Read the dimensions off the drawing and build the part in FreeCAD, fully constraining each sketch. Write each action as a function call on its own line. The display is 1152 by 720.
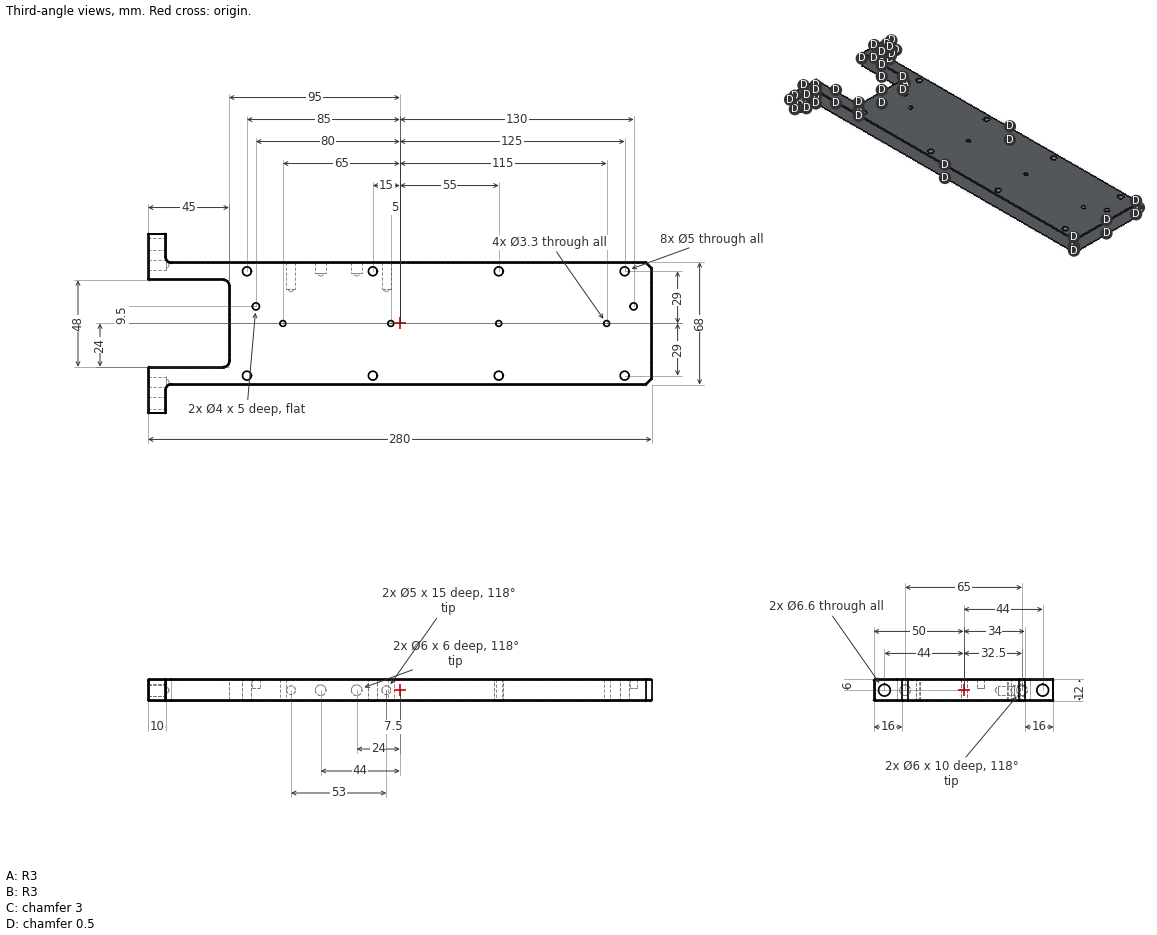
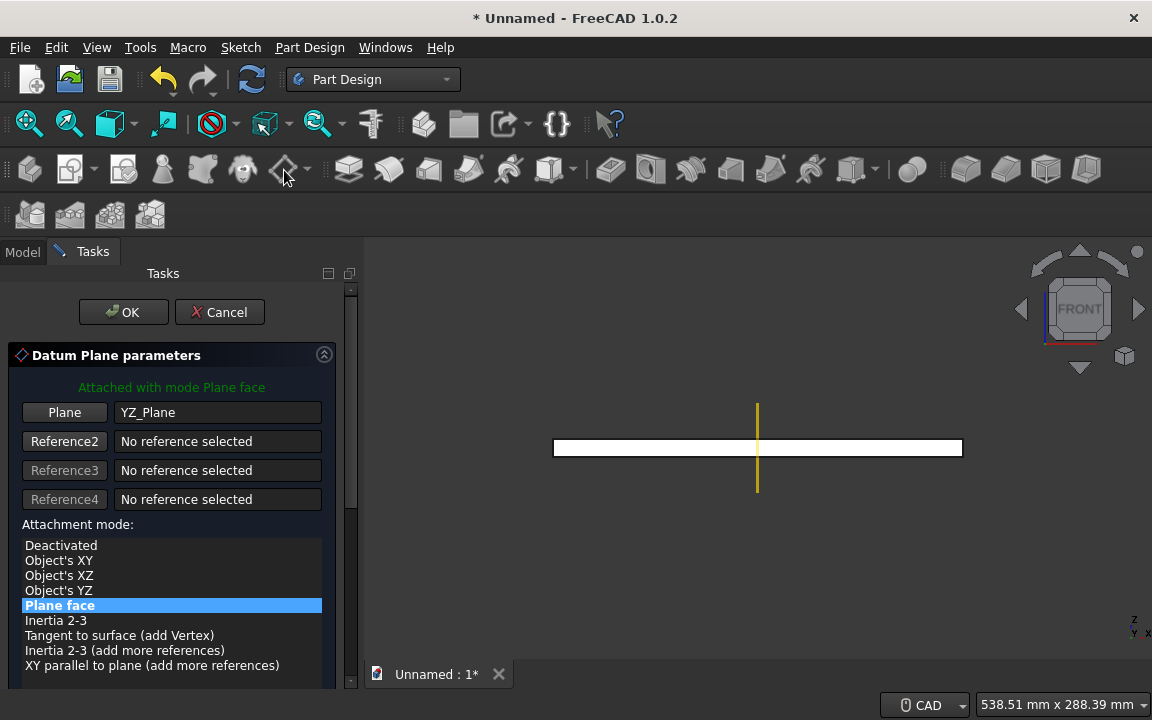
scroll(351, 486, down, 4)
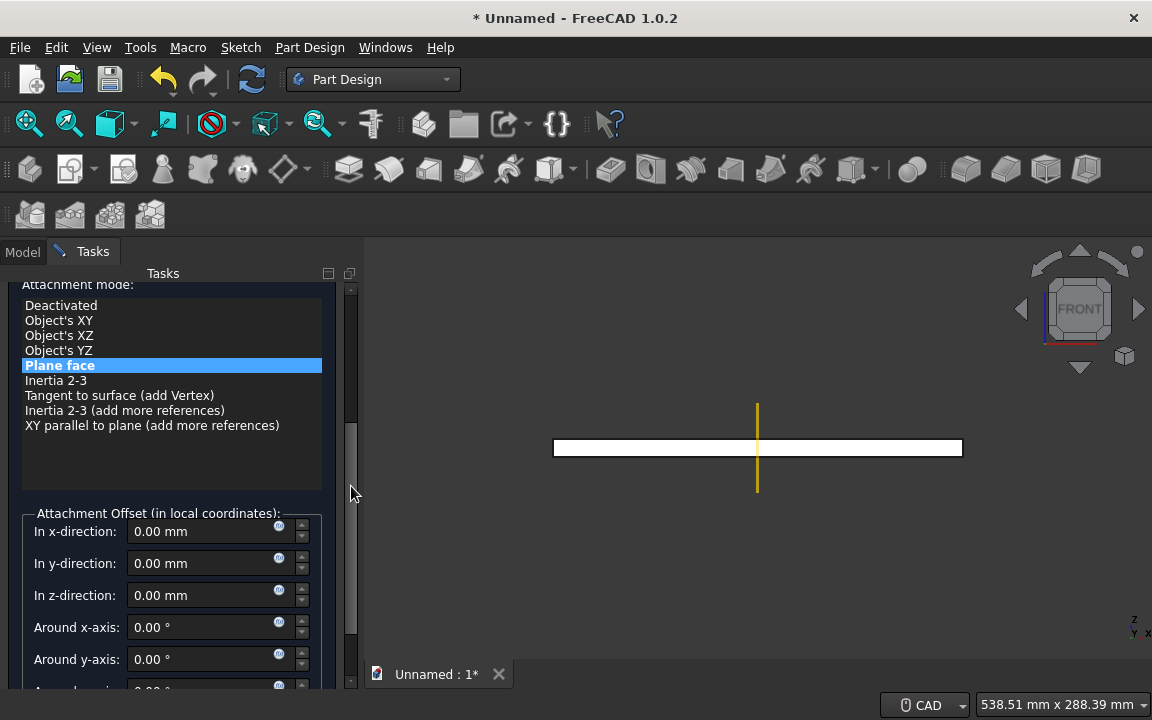
triple_click(210, 595)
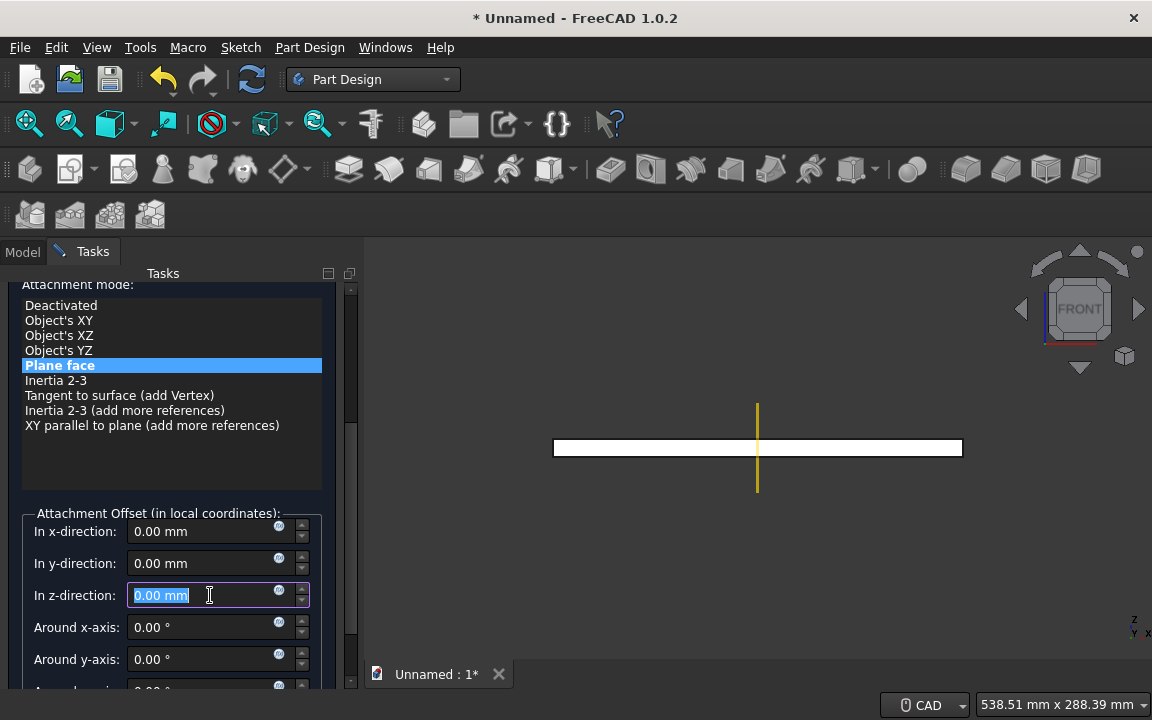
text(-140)
key(Tab)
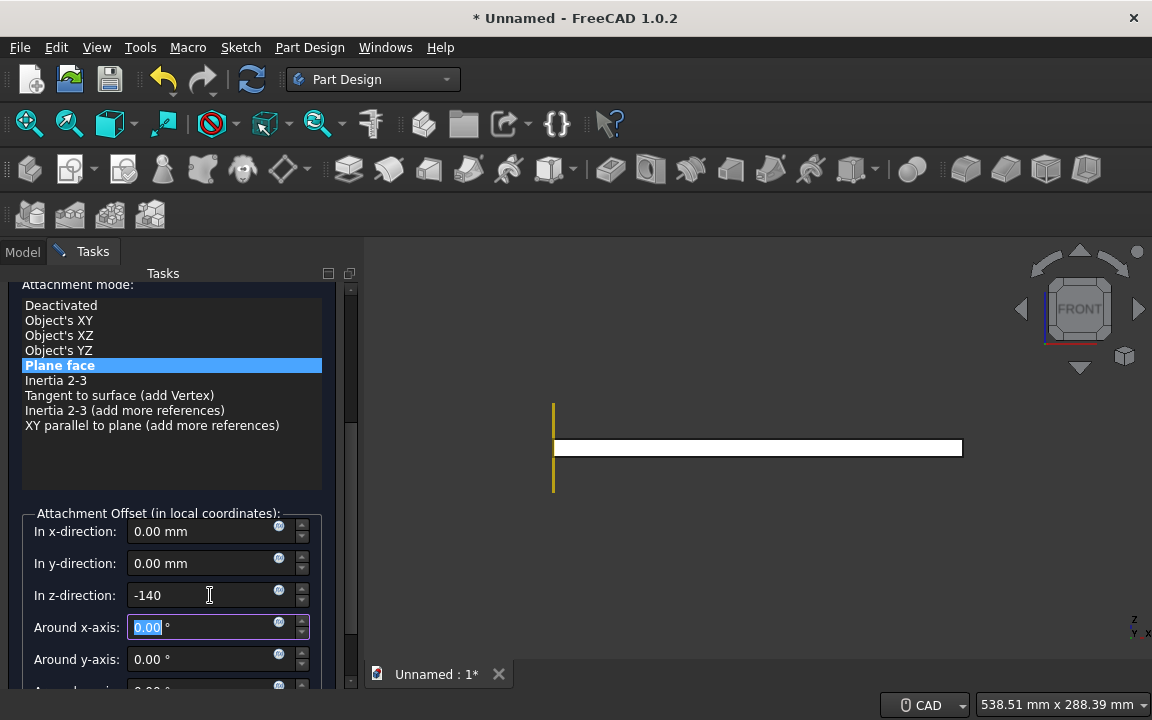
scroll(351, 486, up, 5)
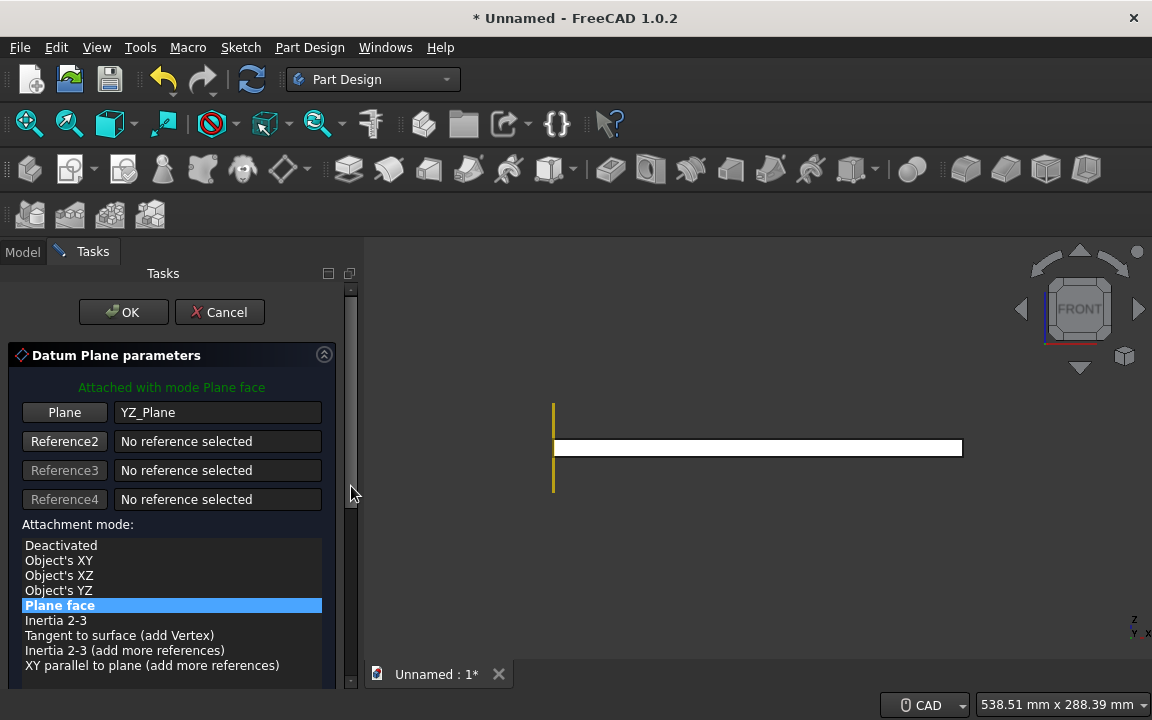
click(124, 312)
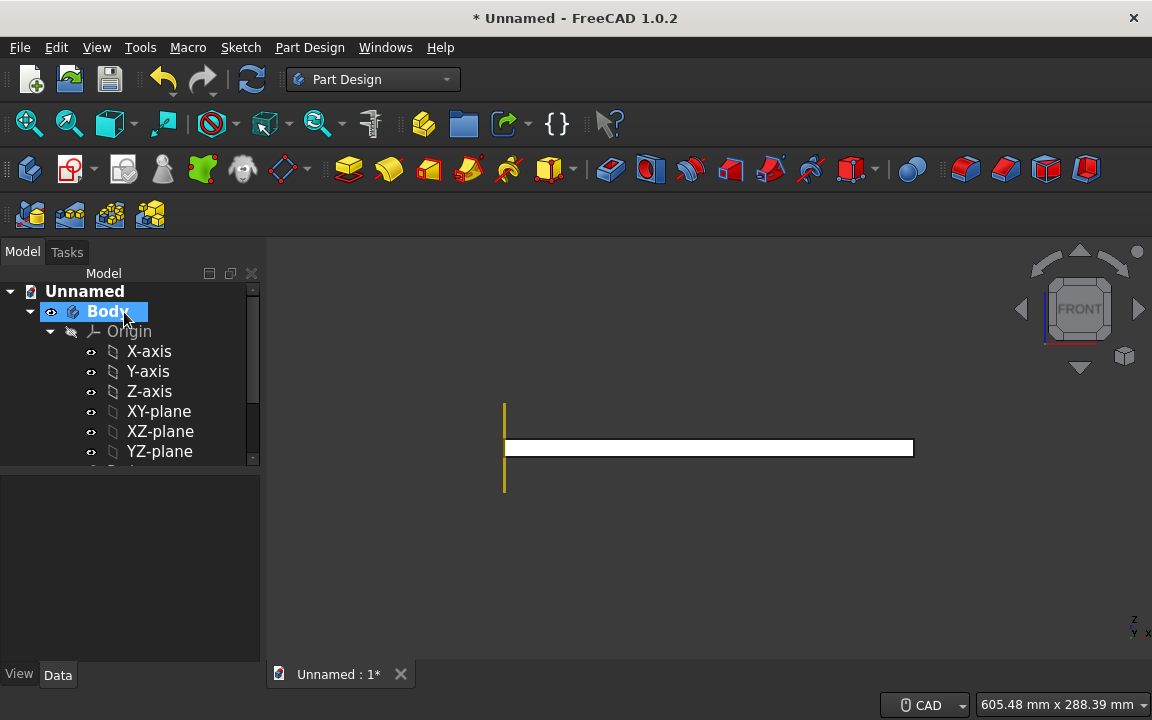
scroll(100, 367, down, 3)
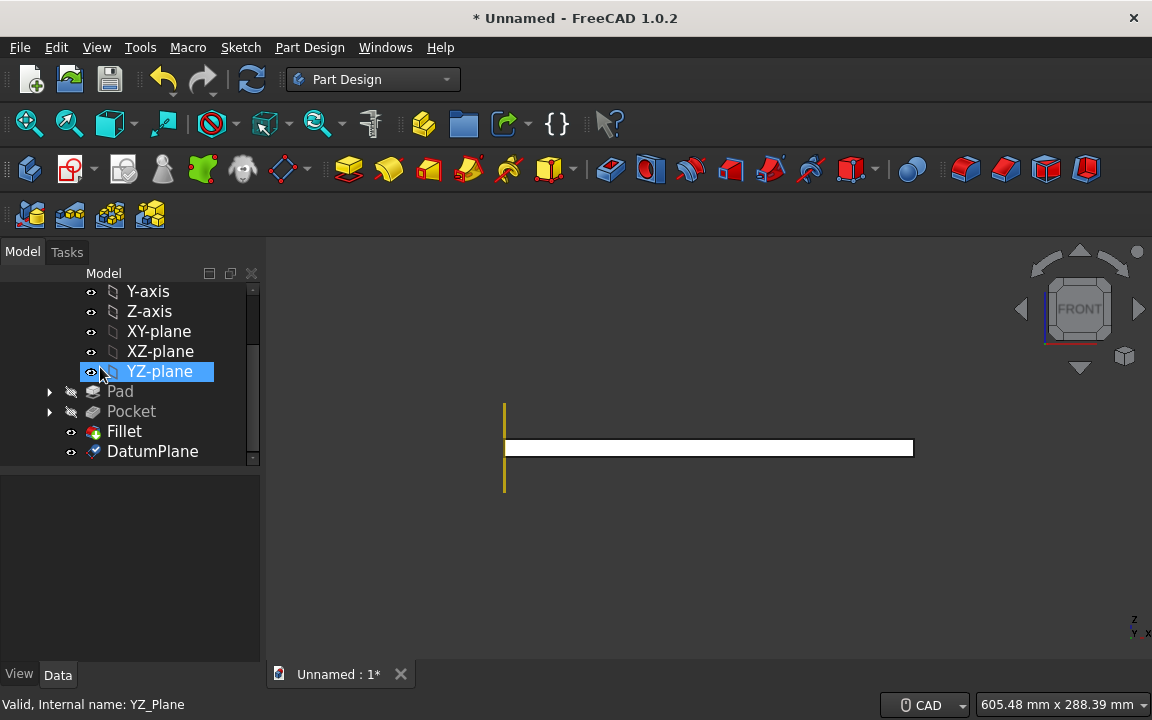
click(116, 452)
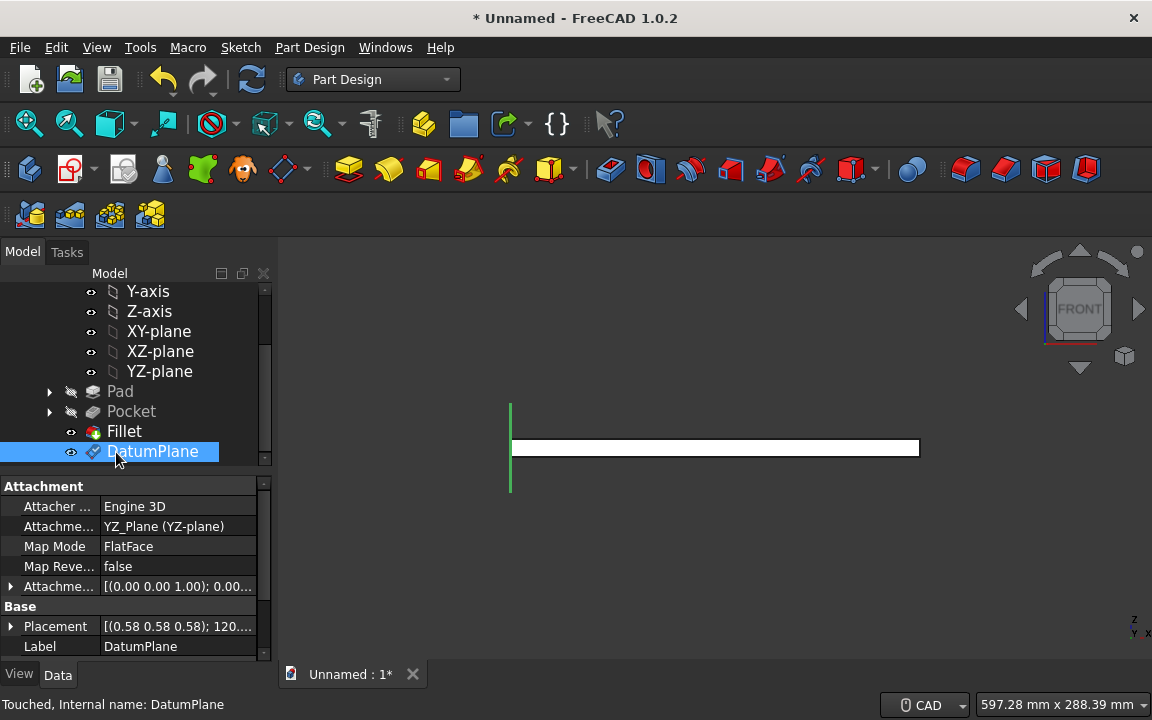
click(70, 170)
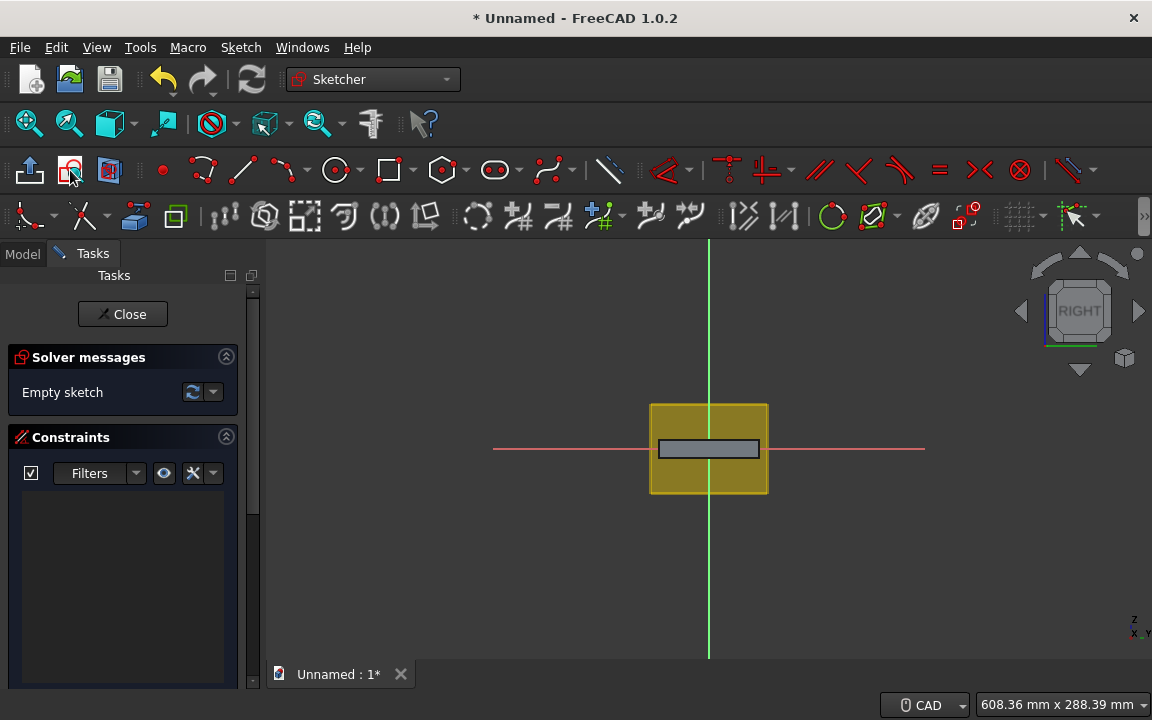
click(110, 170)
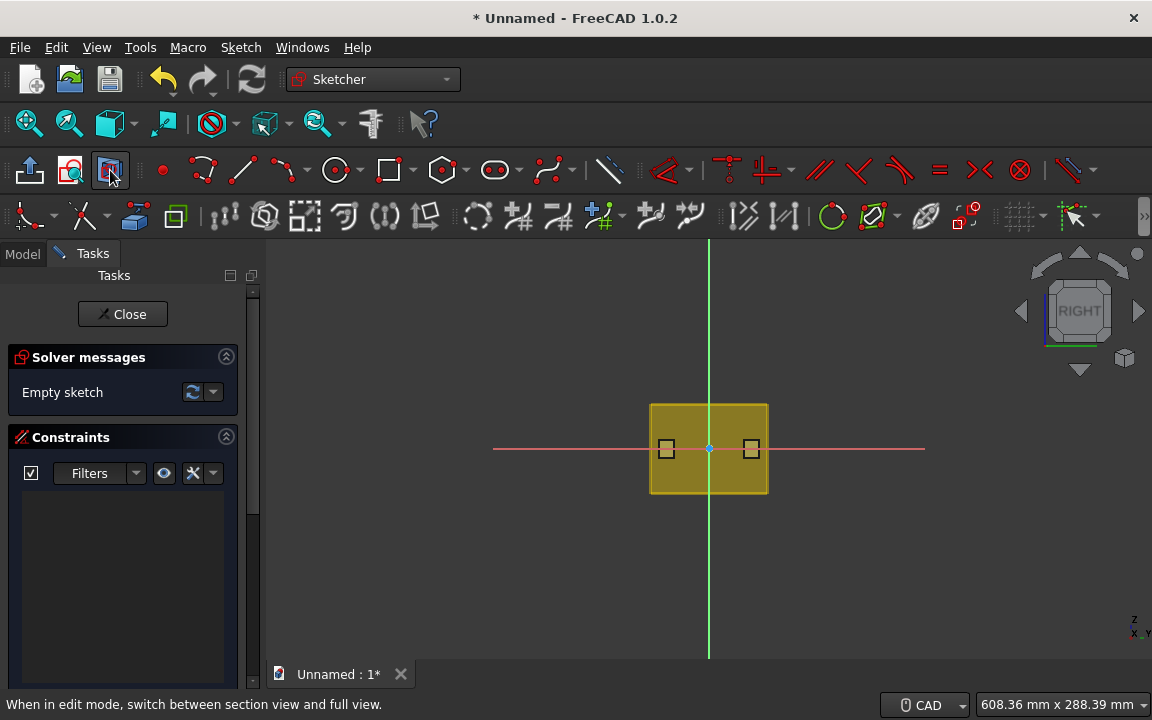
scroll(739, 449, up, 6)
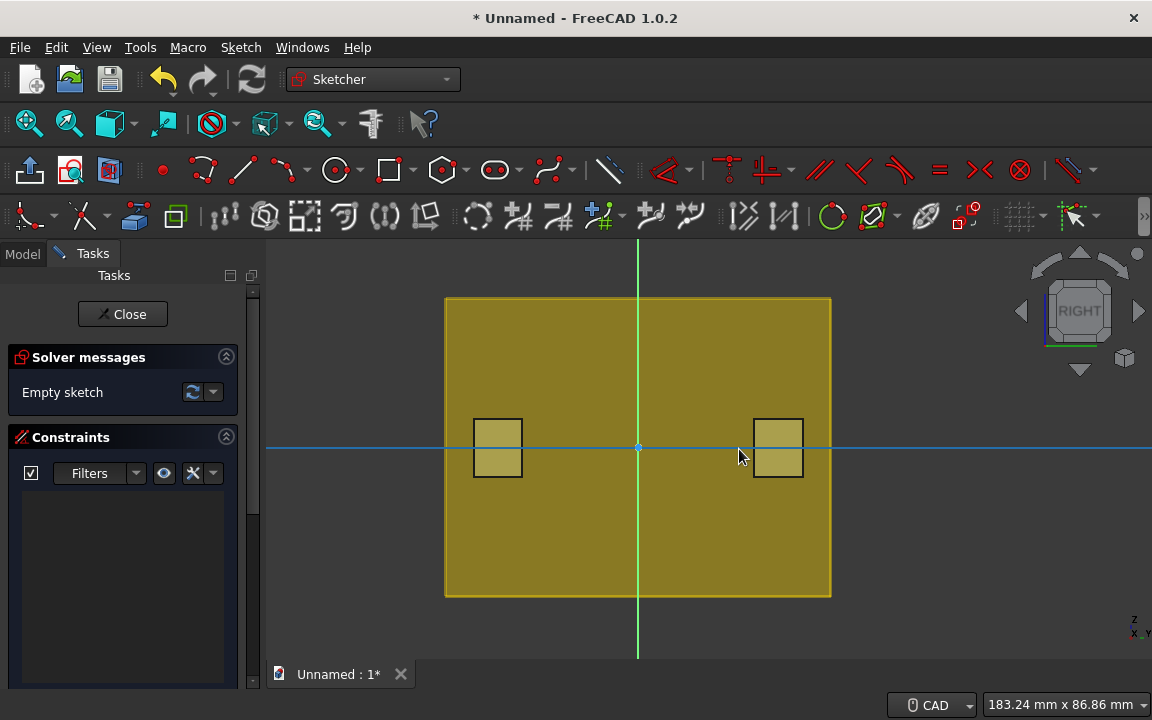
key(g)
key(r)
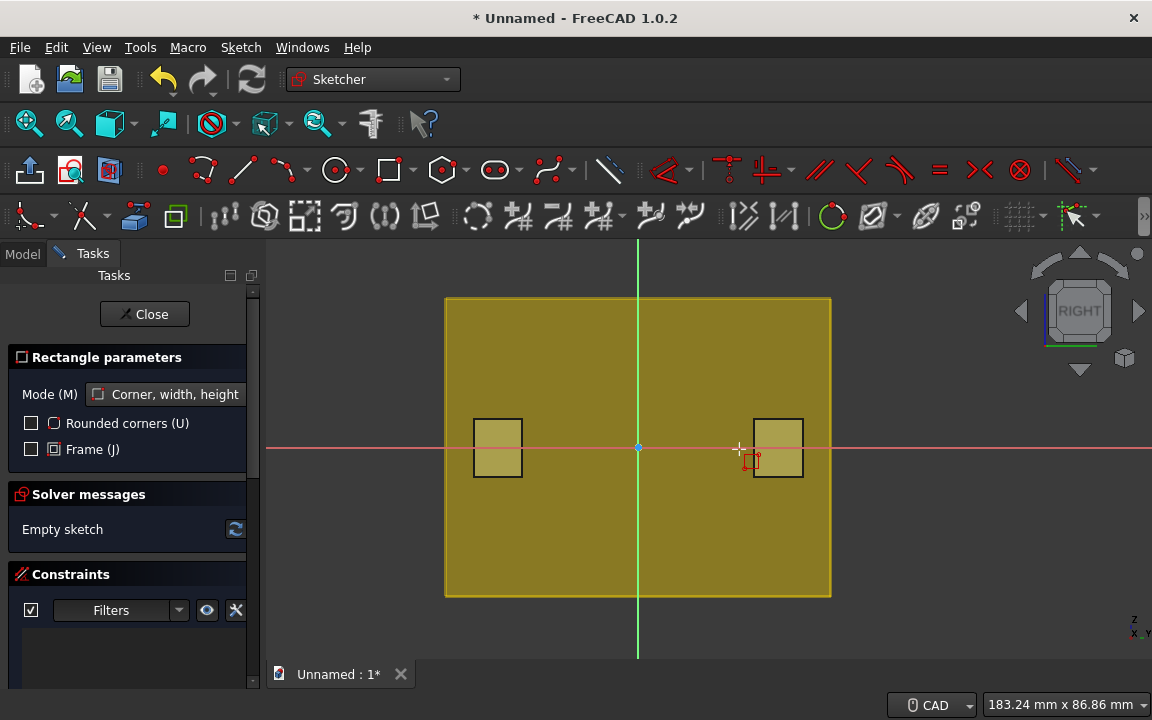
click(396, 419)
move(474, 477)